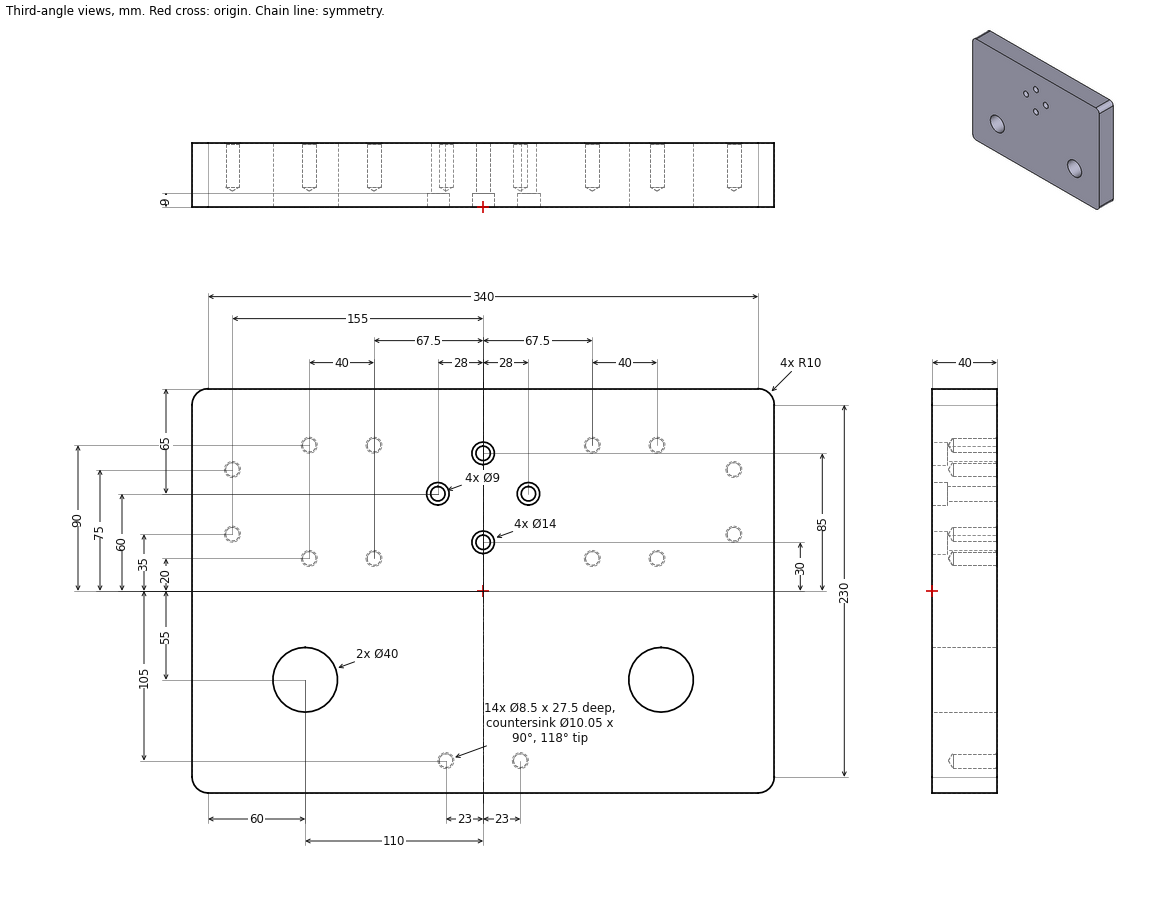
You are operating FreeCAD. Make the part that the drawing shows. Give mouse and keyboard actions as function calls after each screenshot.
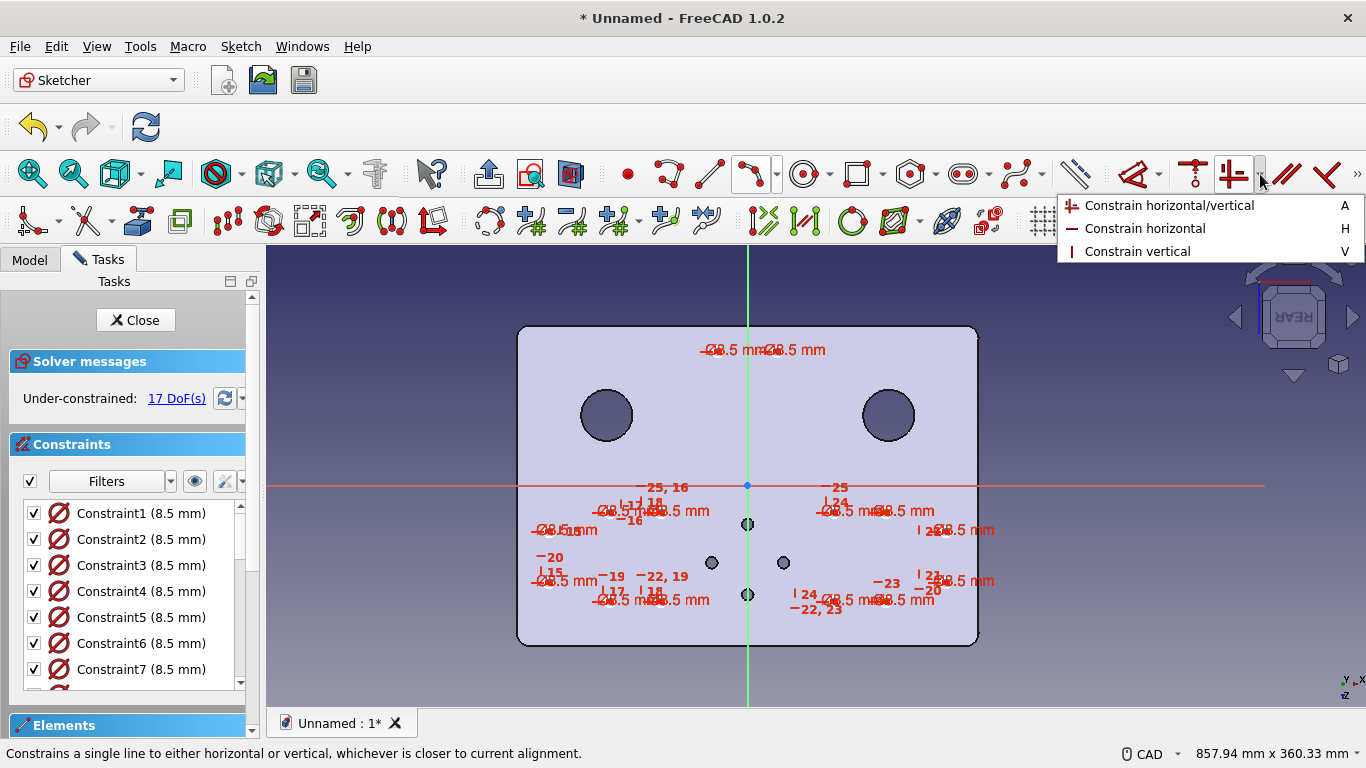
click(1211, 252)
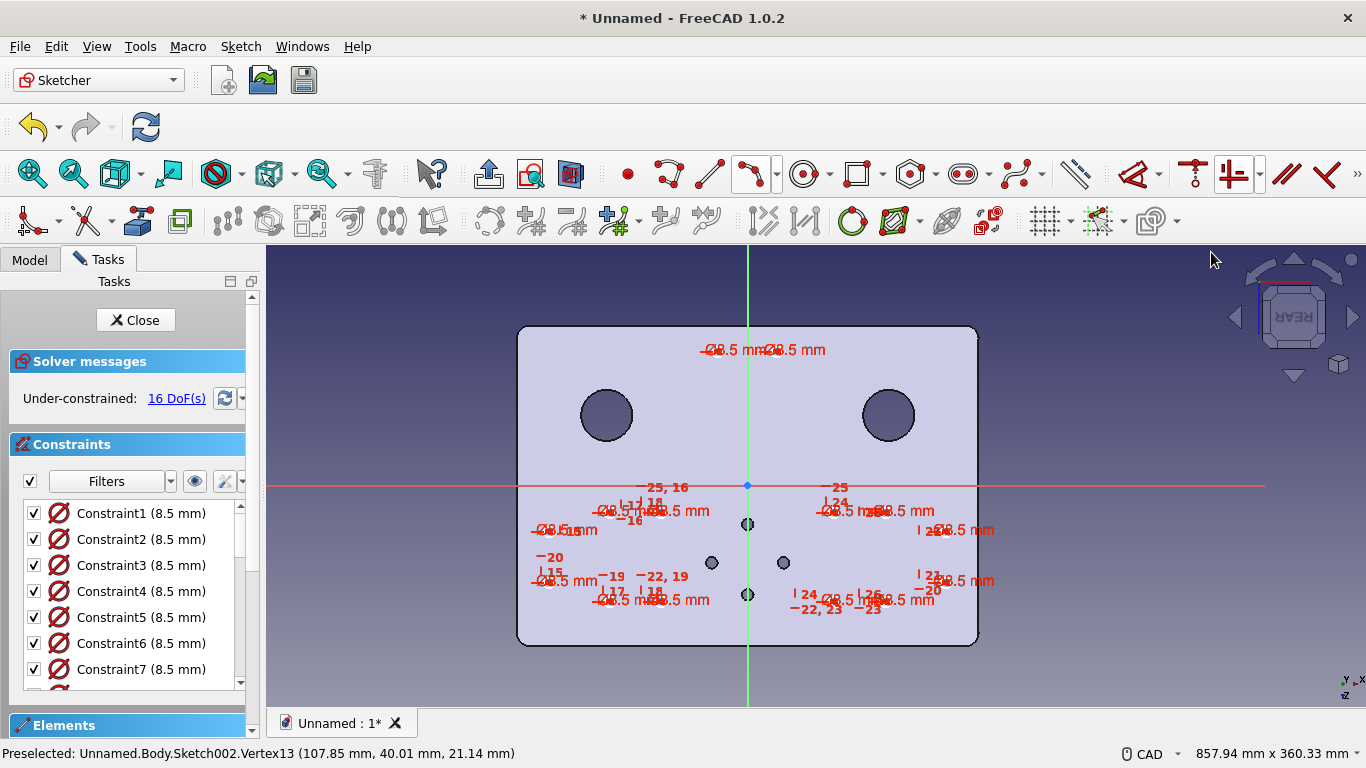
click(834, 513)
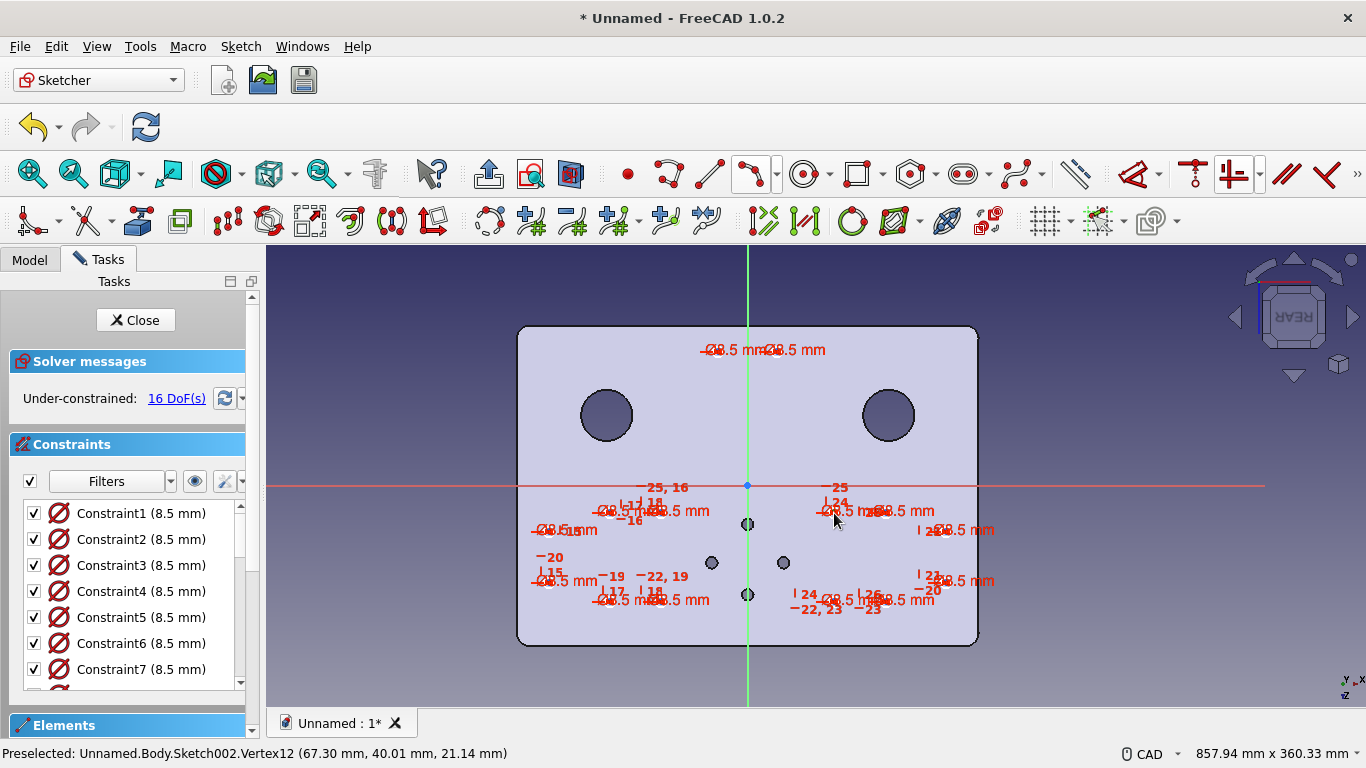
click(886, 513)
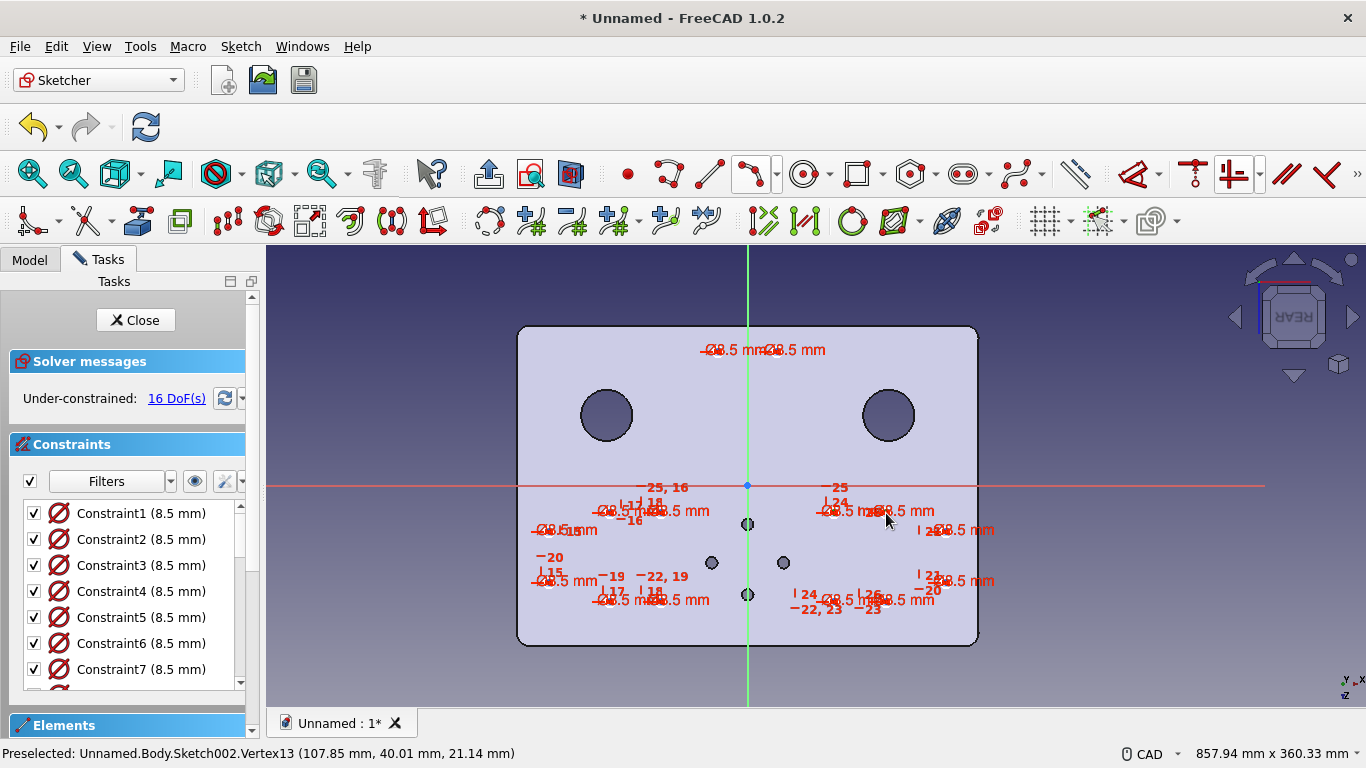
key(h)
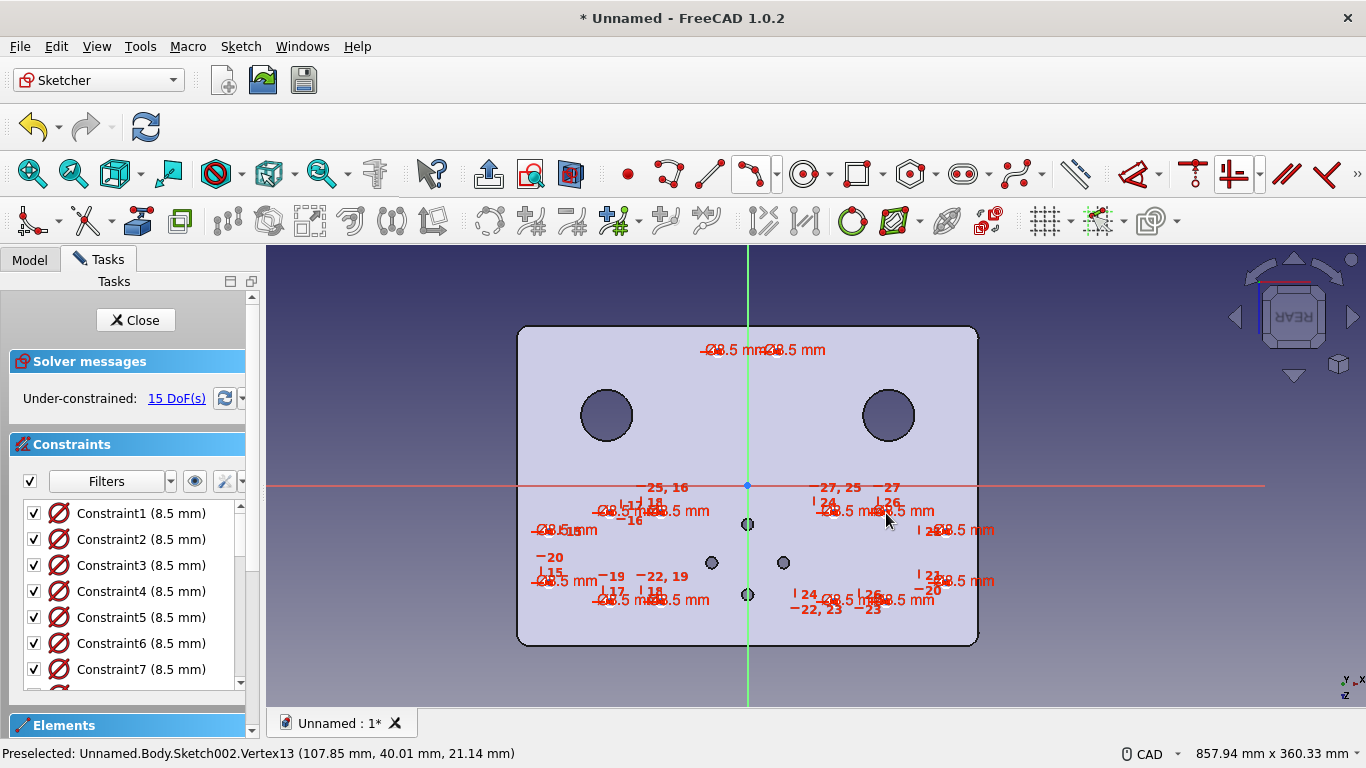
click(718, 352)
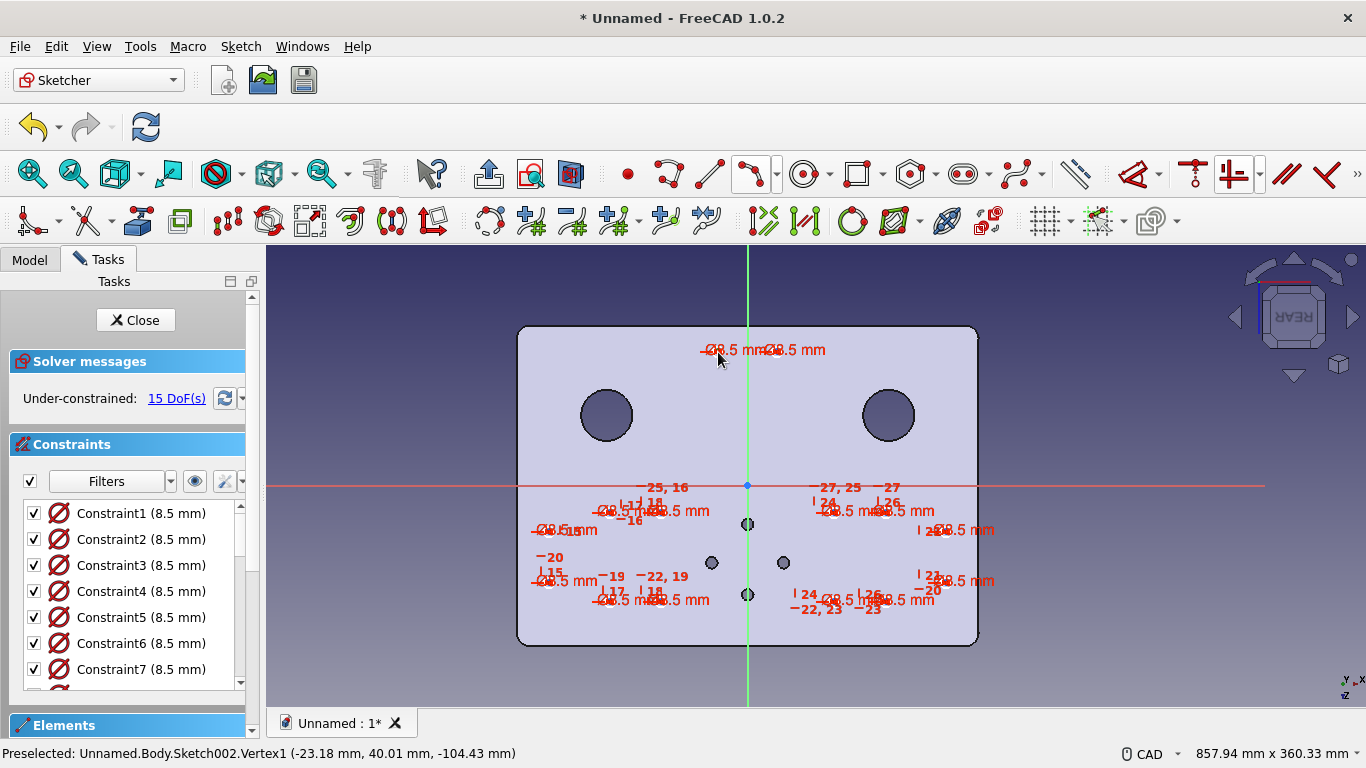
click(777, 352)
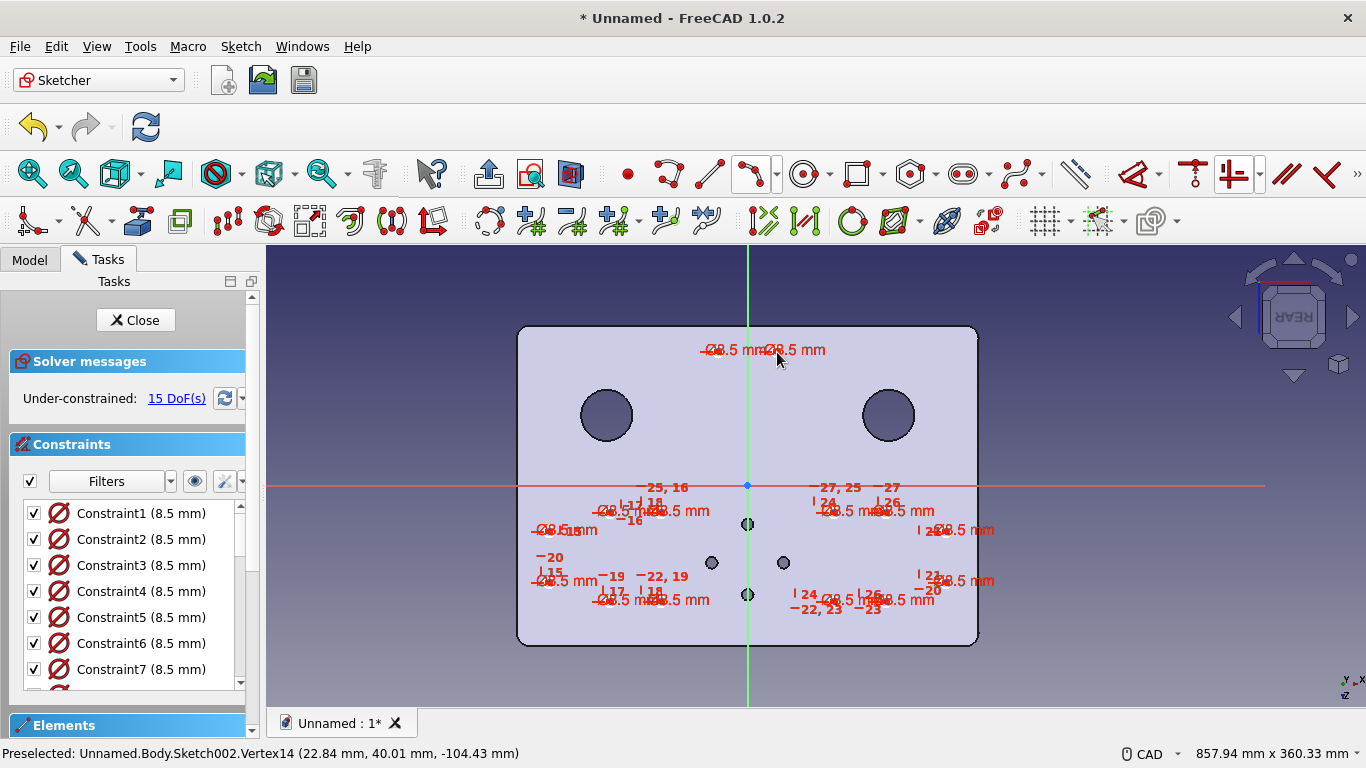
key(h)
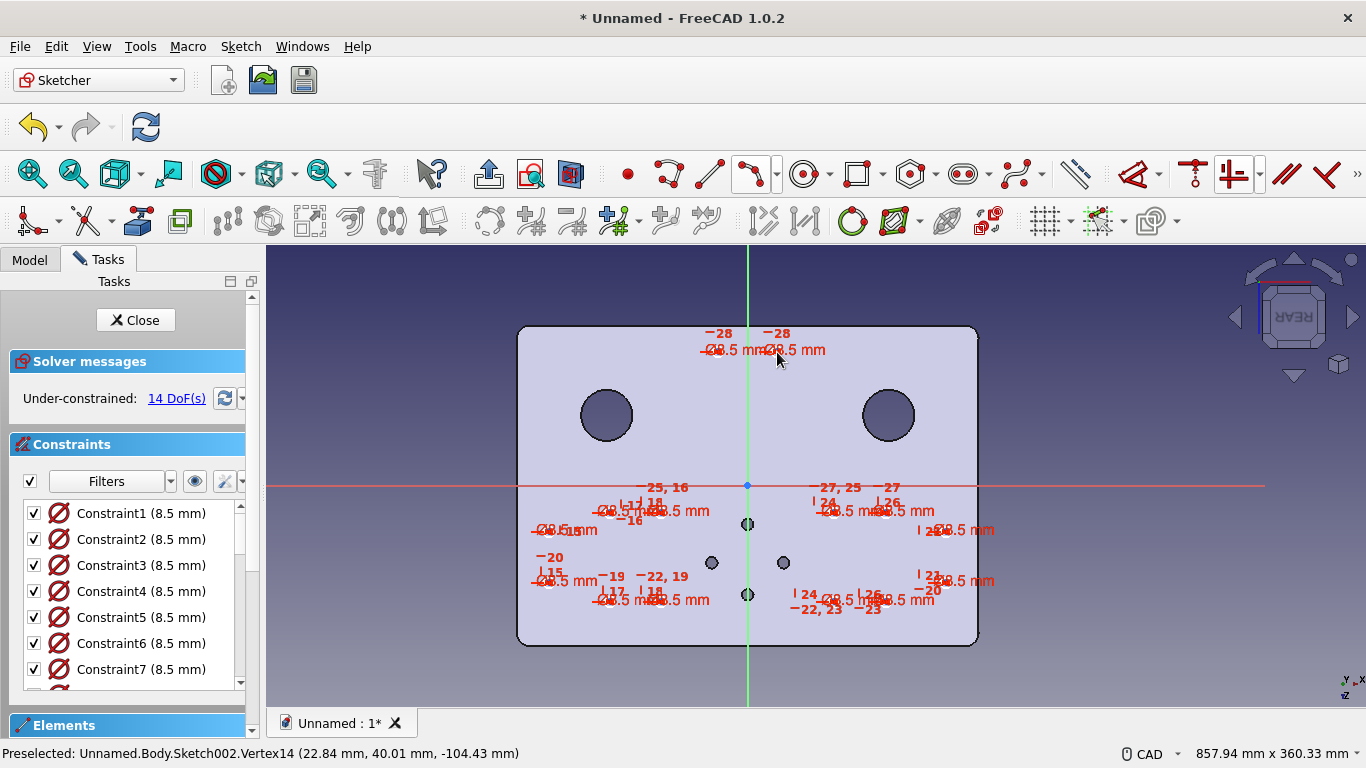
click(549, 532)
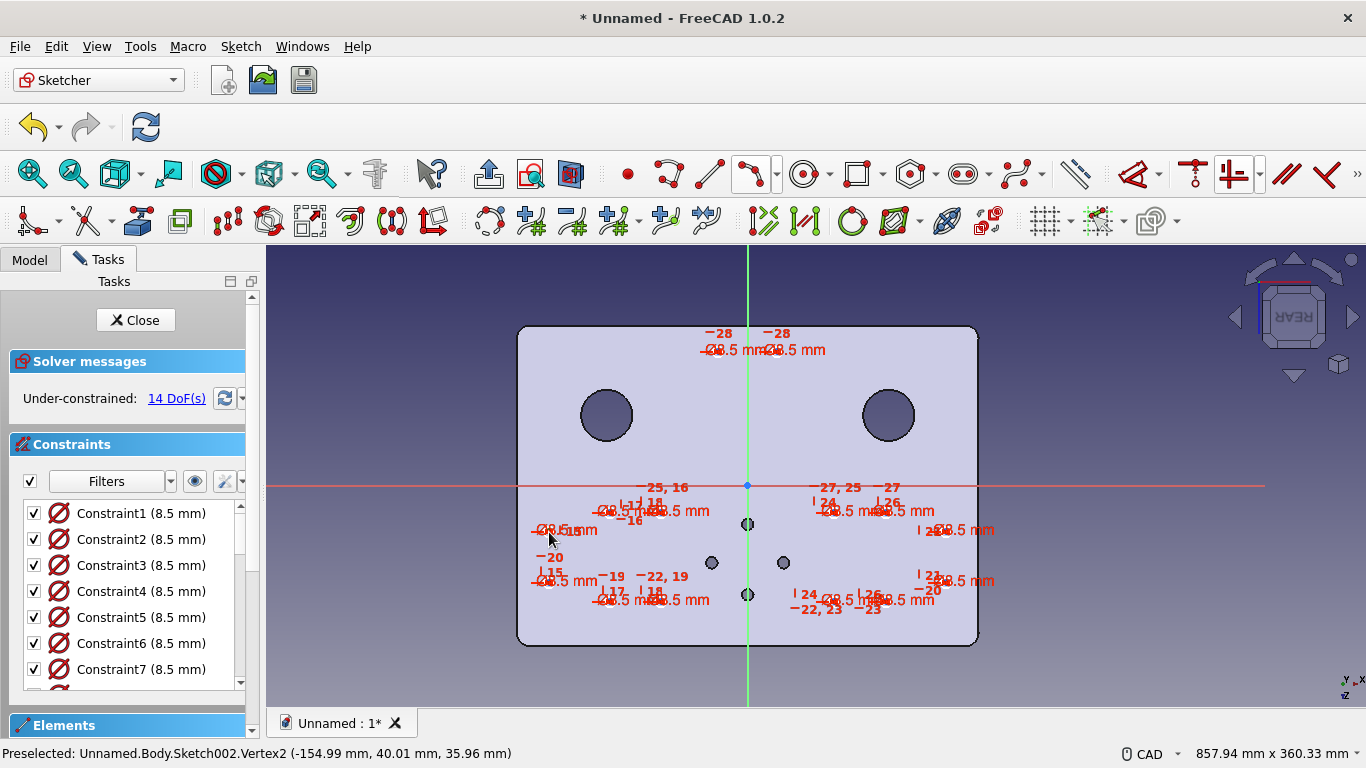
click(946, 532)